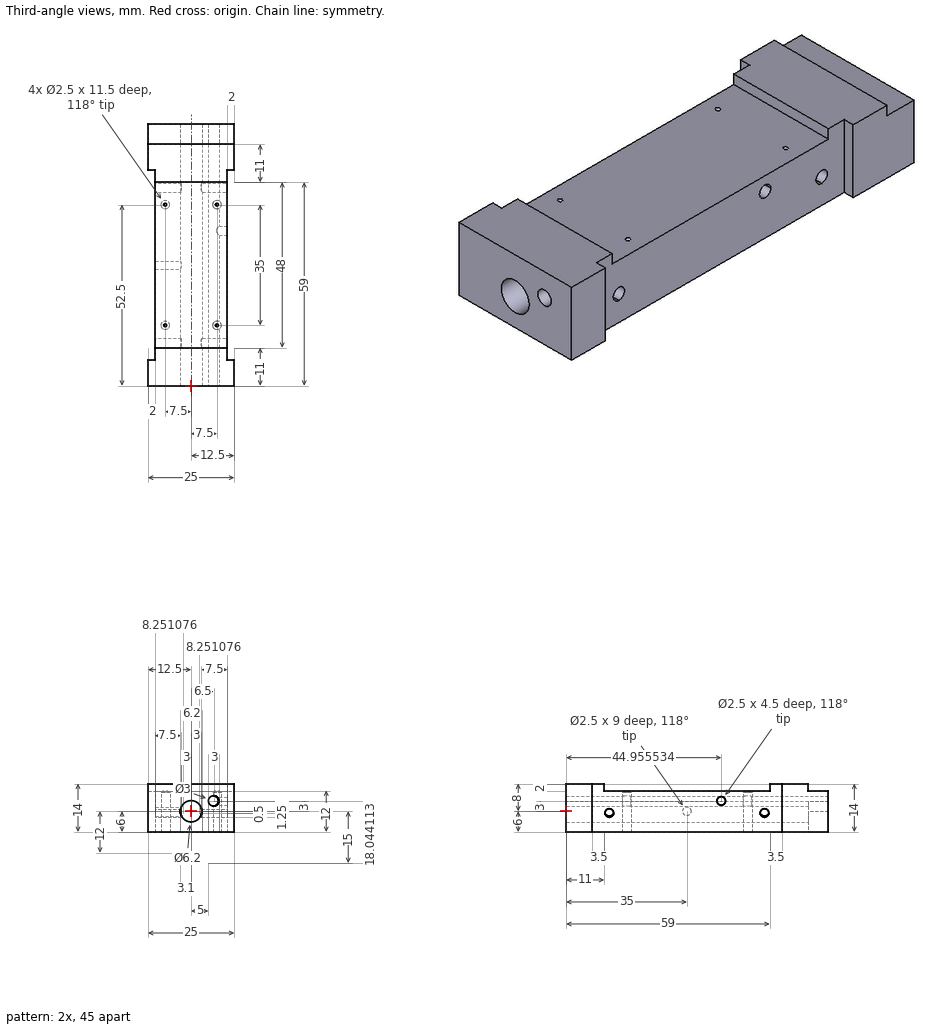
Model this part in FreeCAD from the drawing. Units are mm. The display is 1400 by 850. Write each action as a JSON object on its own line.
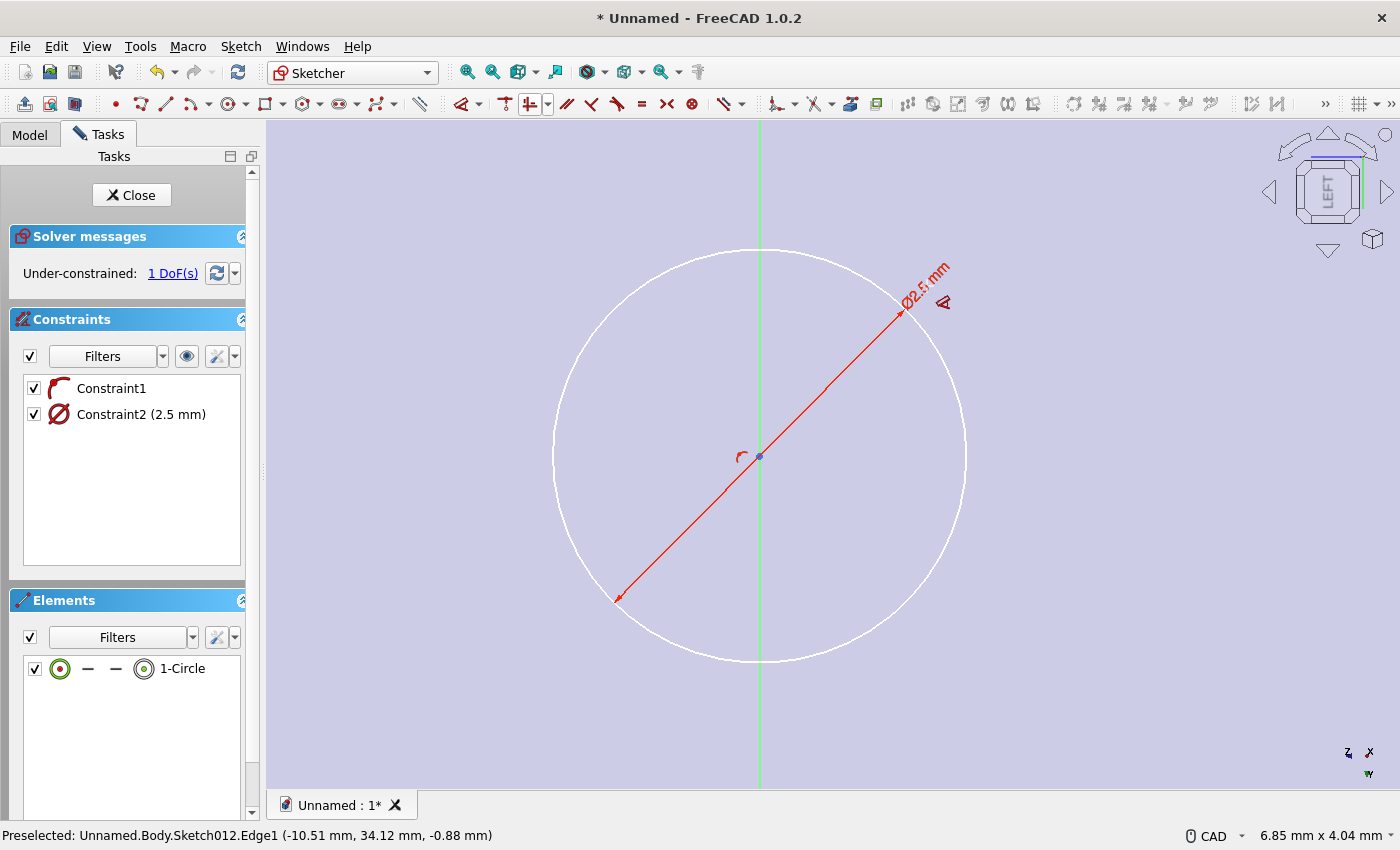
{"action": "left_click", "coordinate": [760, 456]}
{"action": "left_click", "coordinate": [794, 302]}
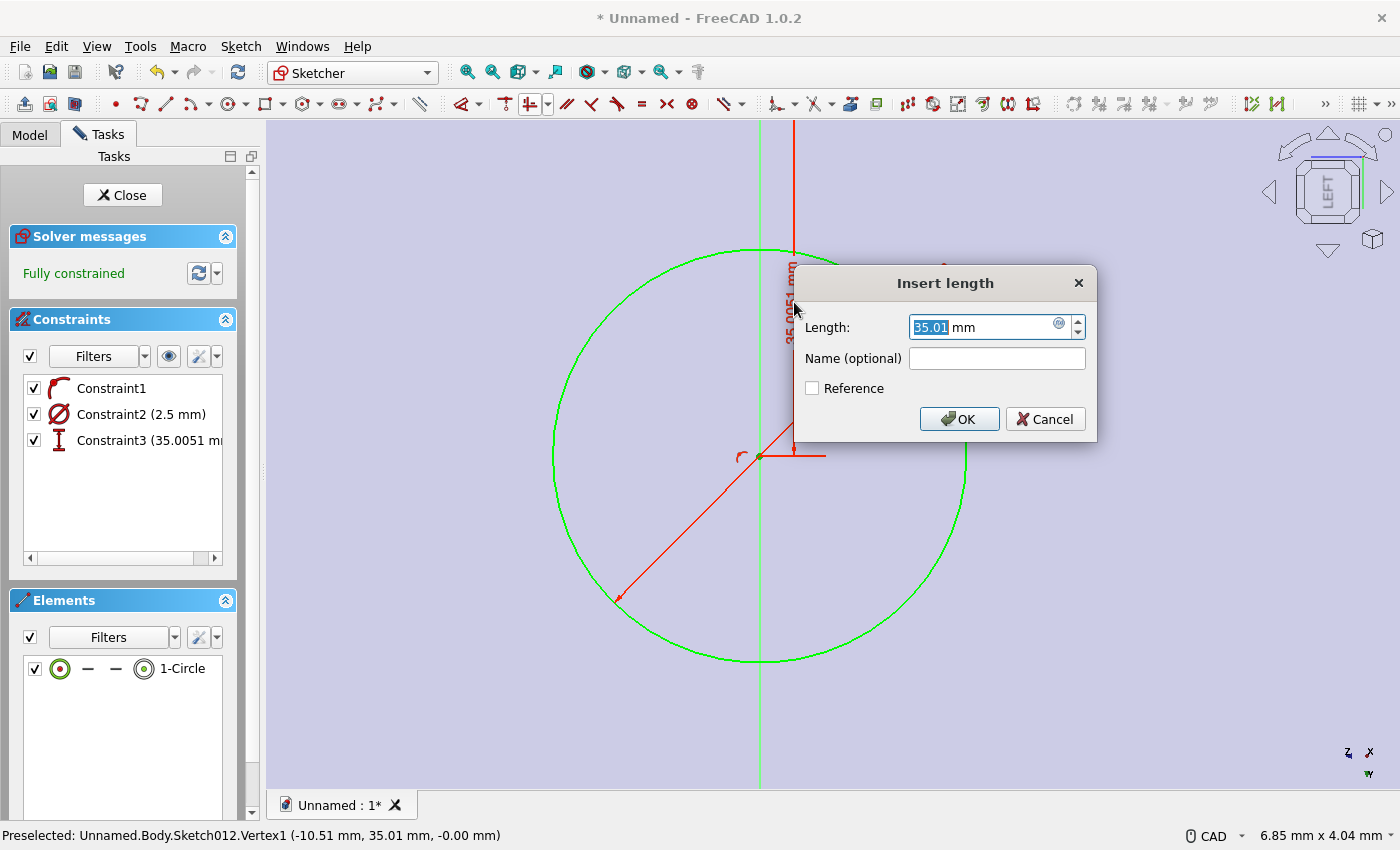
{"action": "type", "text": "35"}
{"action": "key", "text": "Return"}
{"action": "key", "text": "Escape"}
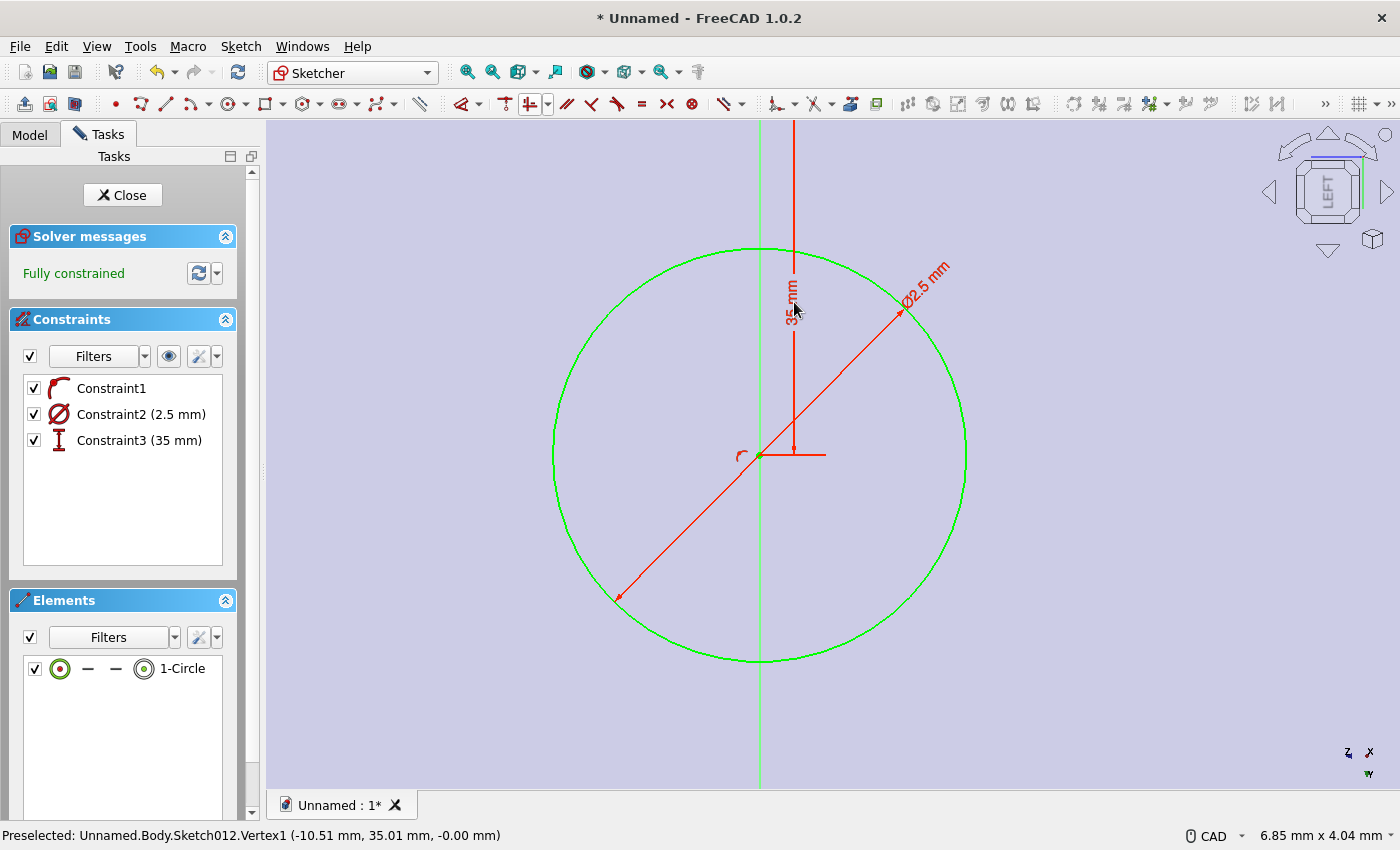
{"action": "left_click", "coordinate": [123, 195]}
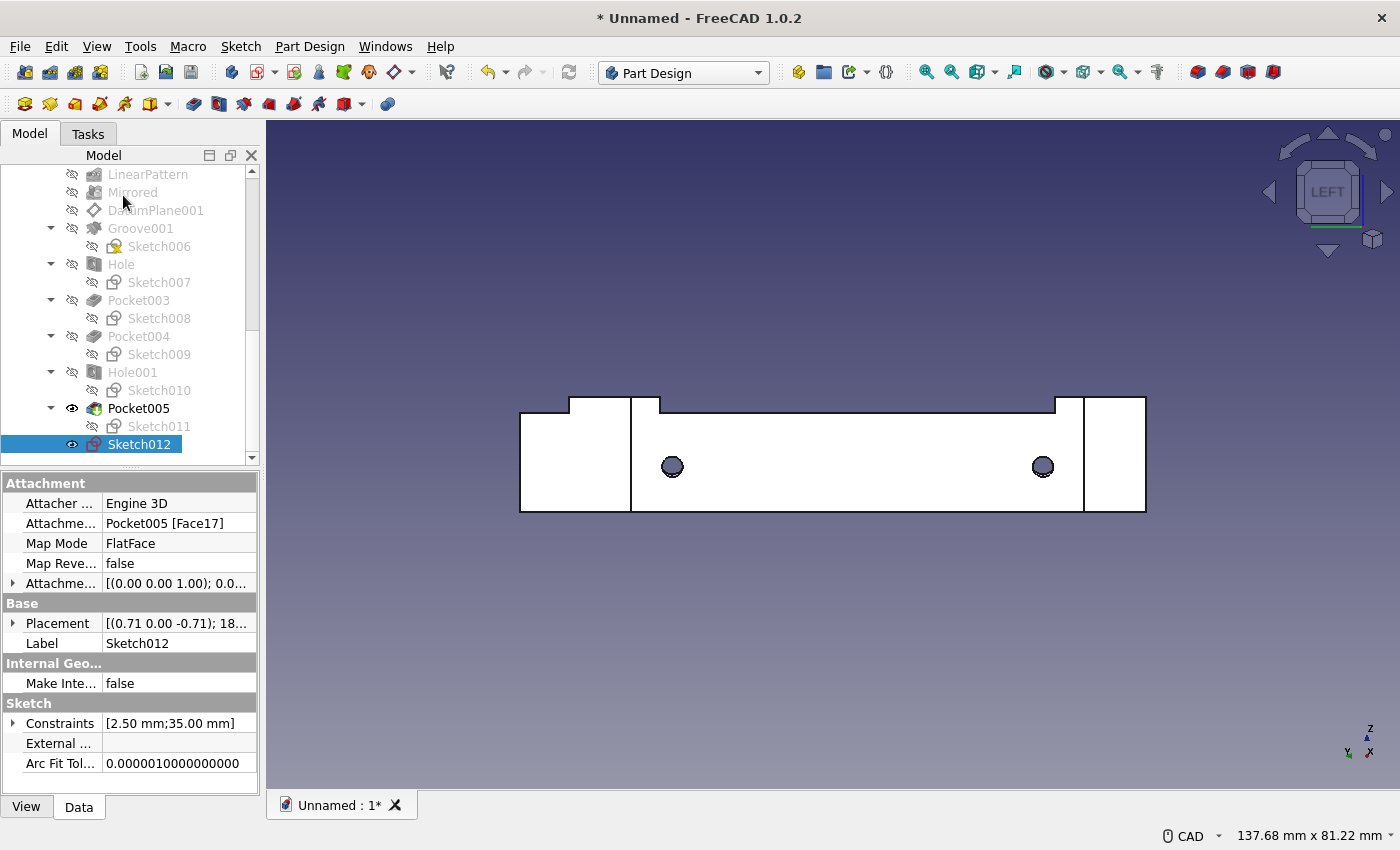
{"action": "left_click", "coordinate": [219, 104]}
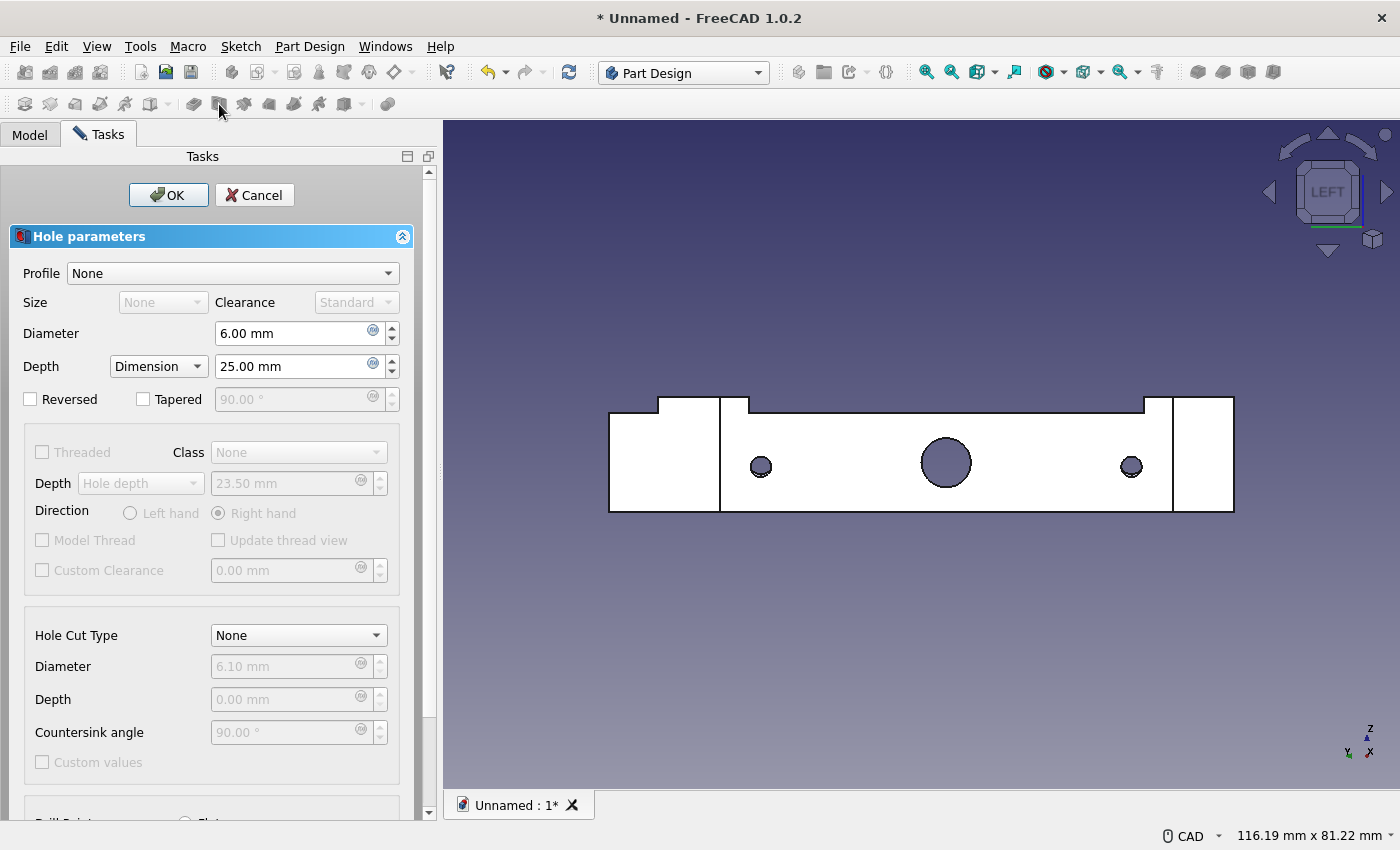
{"action": "triple_click", "coordinate": [300, 334]}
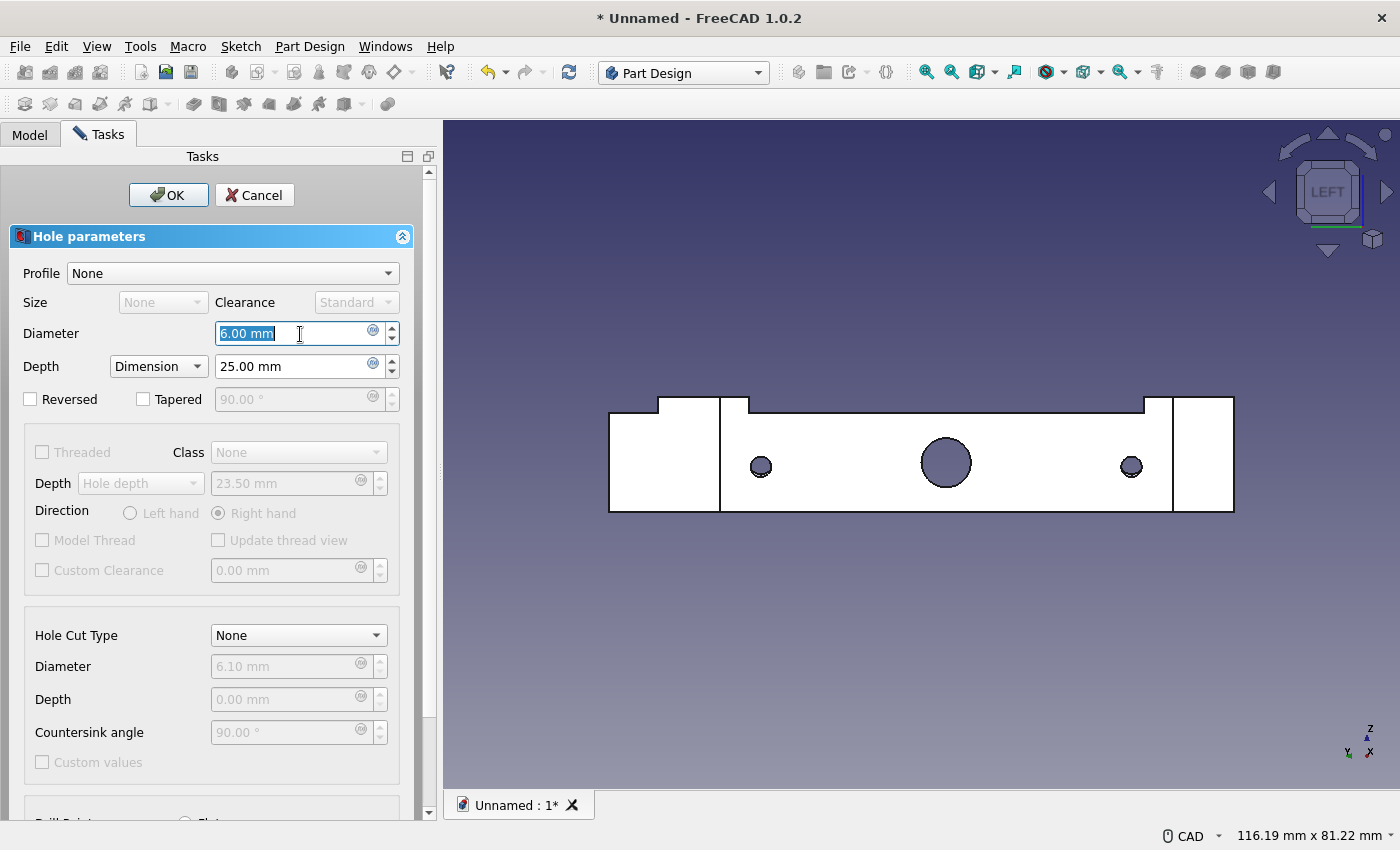
{"action": "type", "text": "2.5"}
{"action": "key", "text": "Tab"}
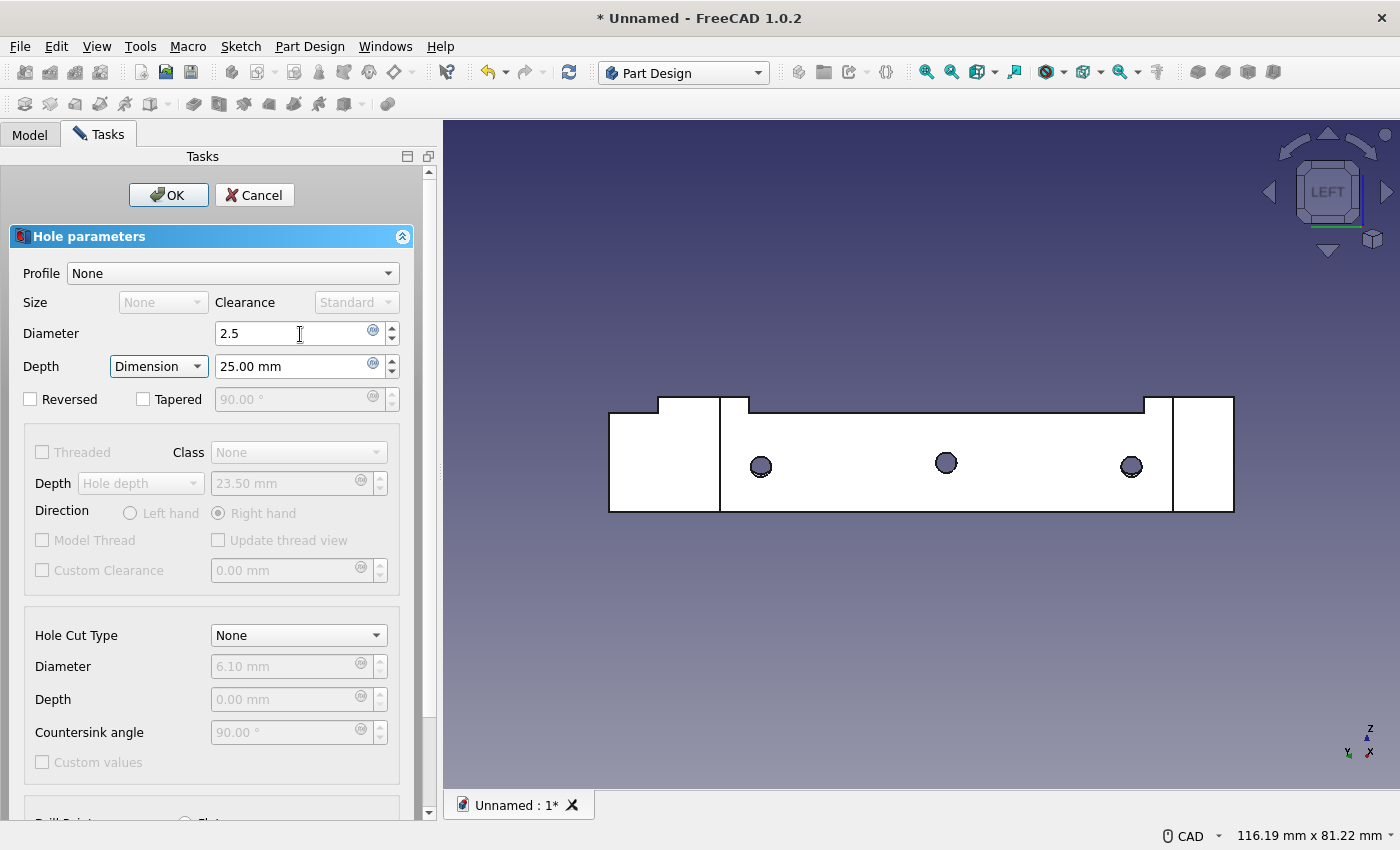
{"action": "triple_click", "coordinate": [300, 366]}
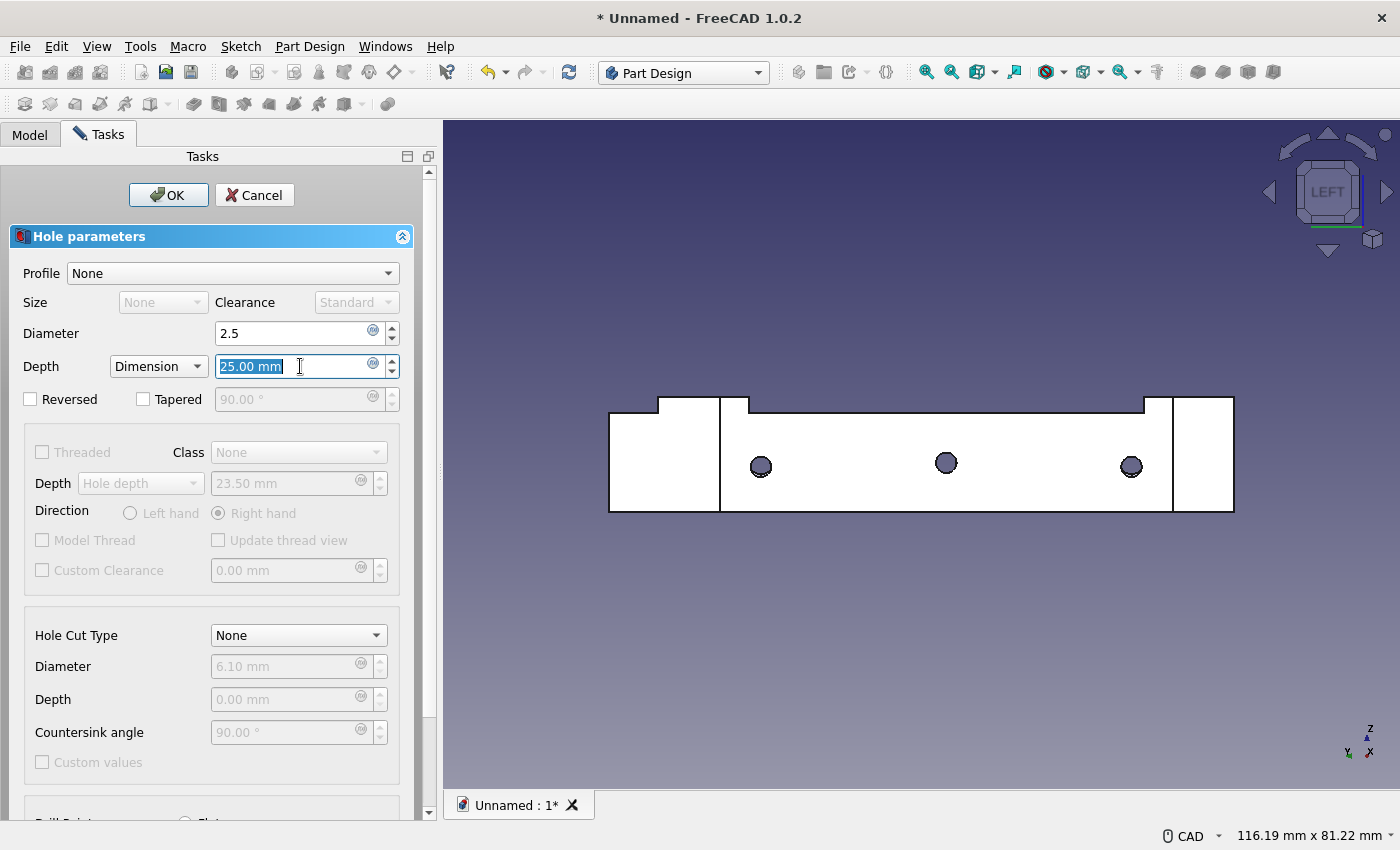
{"action": "type", "text": "9"}
{"action": "key", "text": "Tab"}